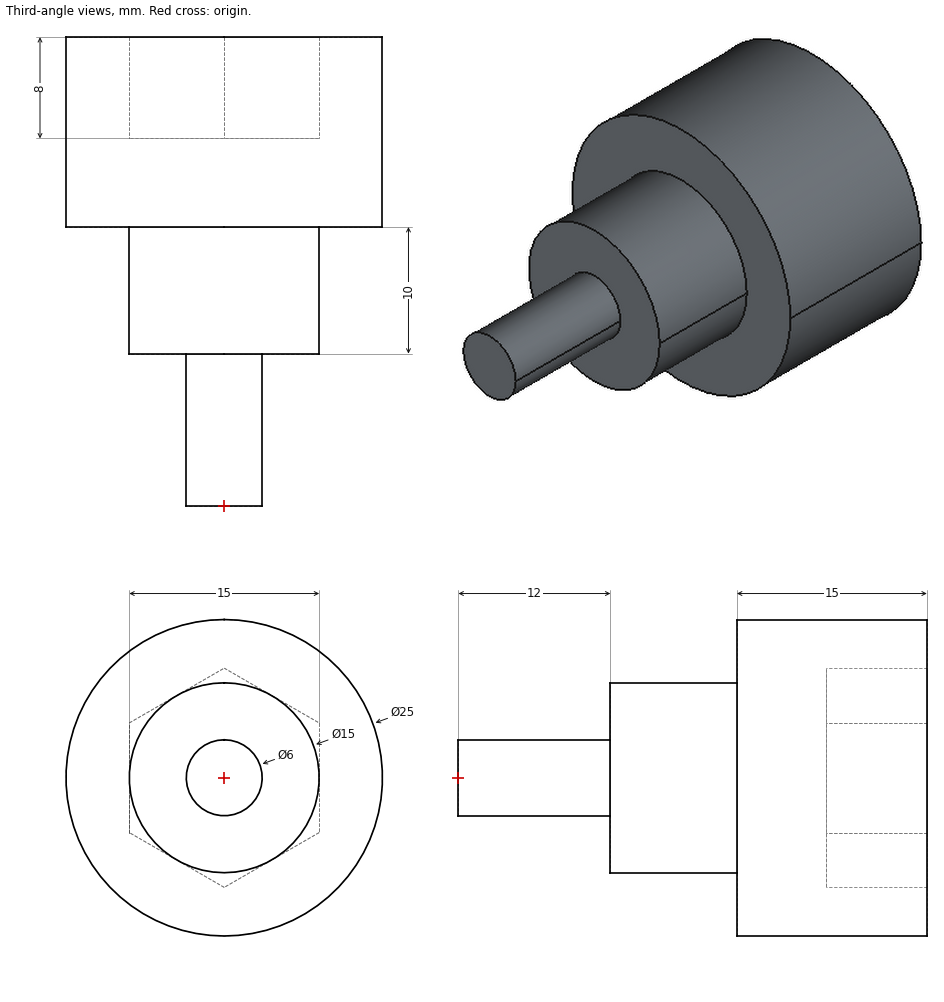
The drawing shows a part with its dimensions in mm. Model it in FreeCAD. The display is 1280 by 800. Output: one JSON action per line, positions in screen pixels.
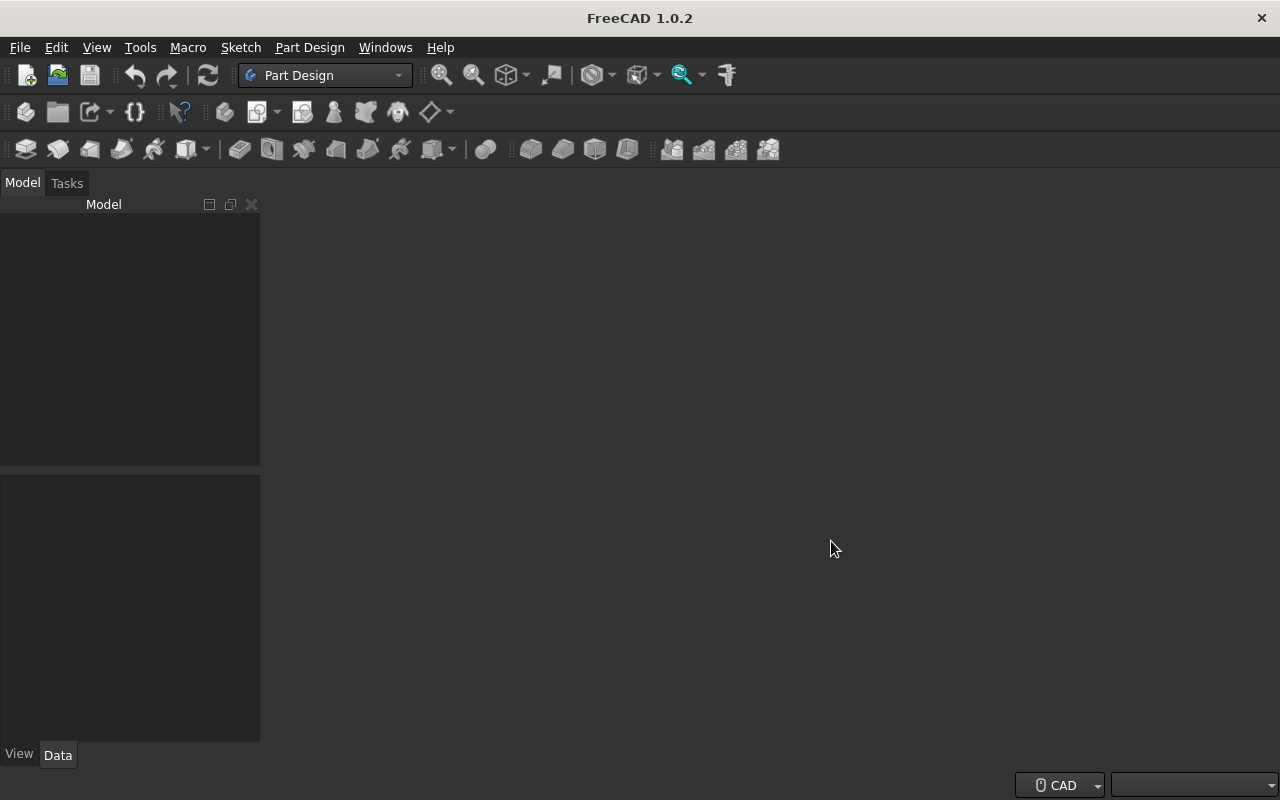
{"action": "key", "text": "ctrl+n"}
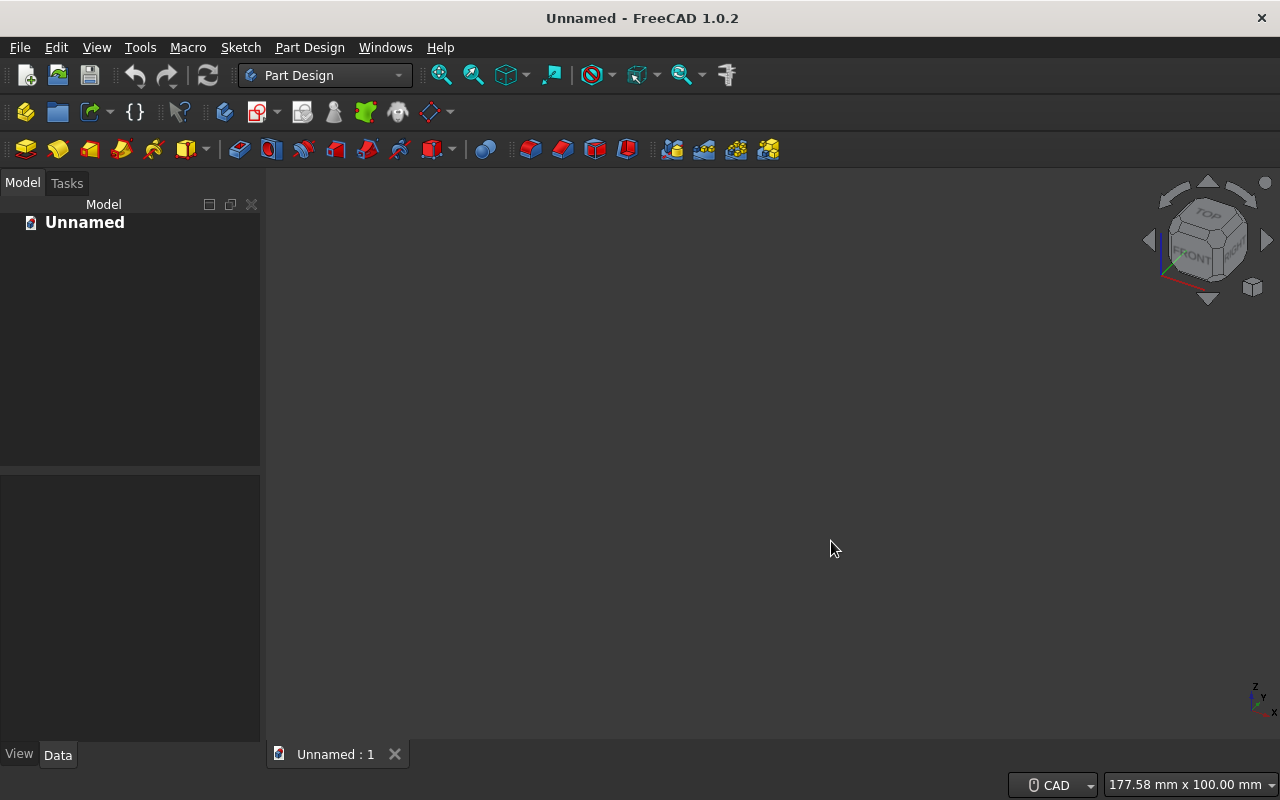
{"action": "left_click", "coordinate": [258, 112]}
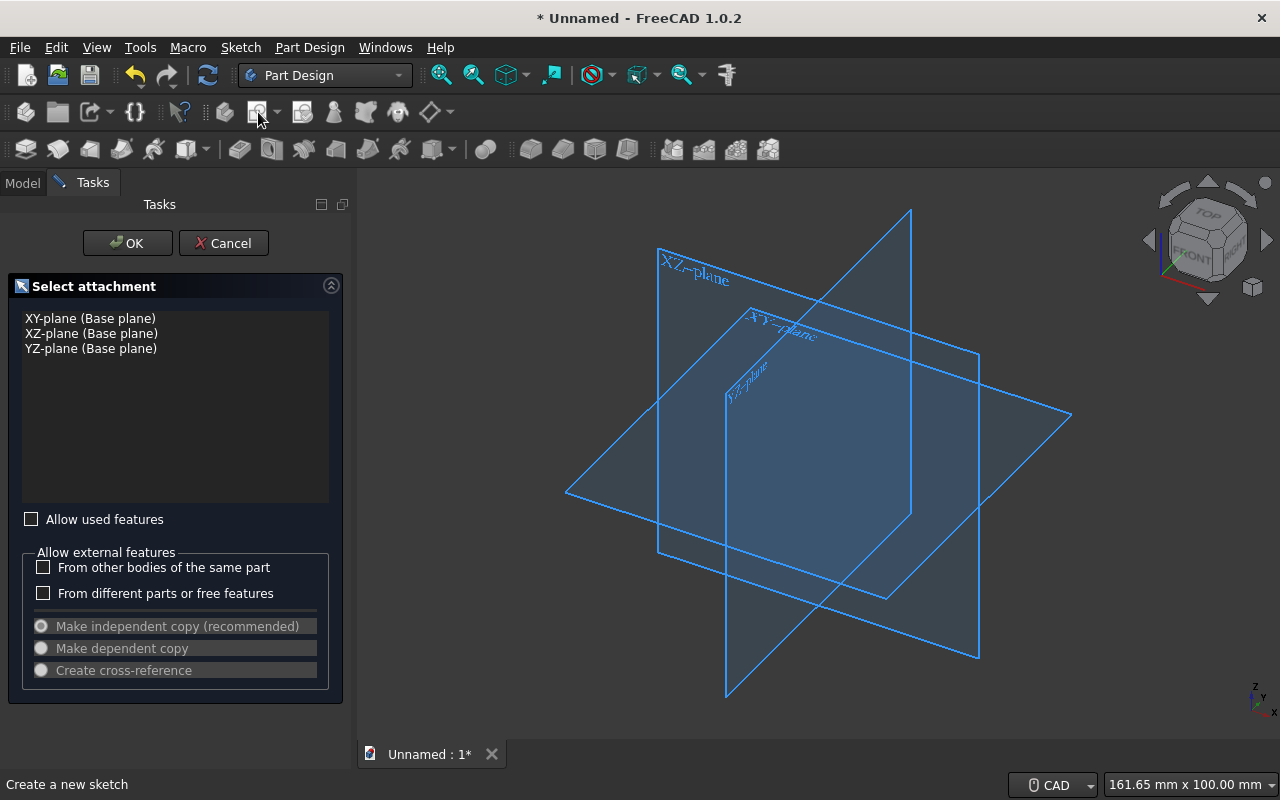
{"action": "left_click", "coordinate": [82, 334]}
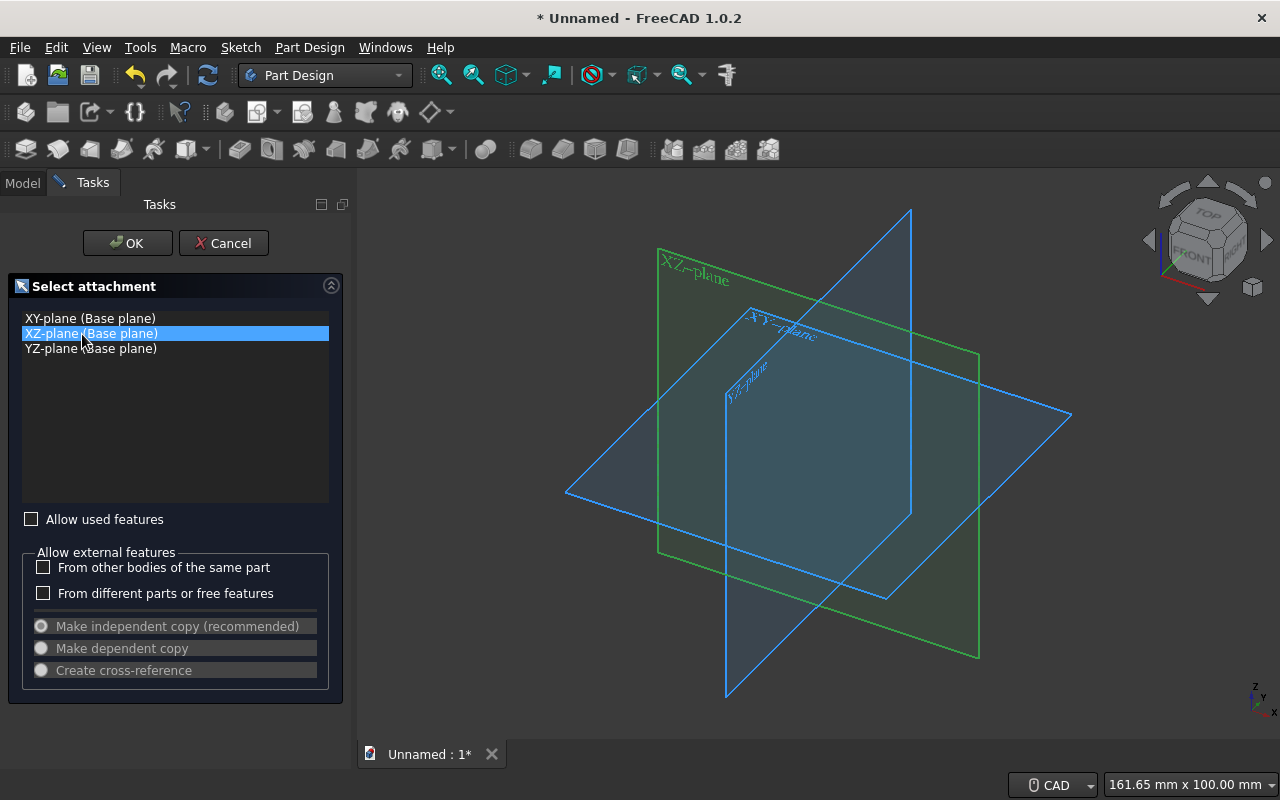
{"action": "left_click", "coordinate": [128, 243]}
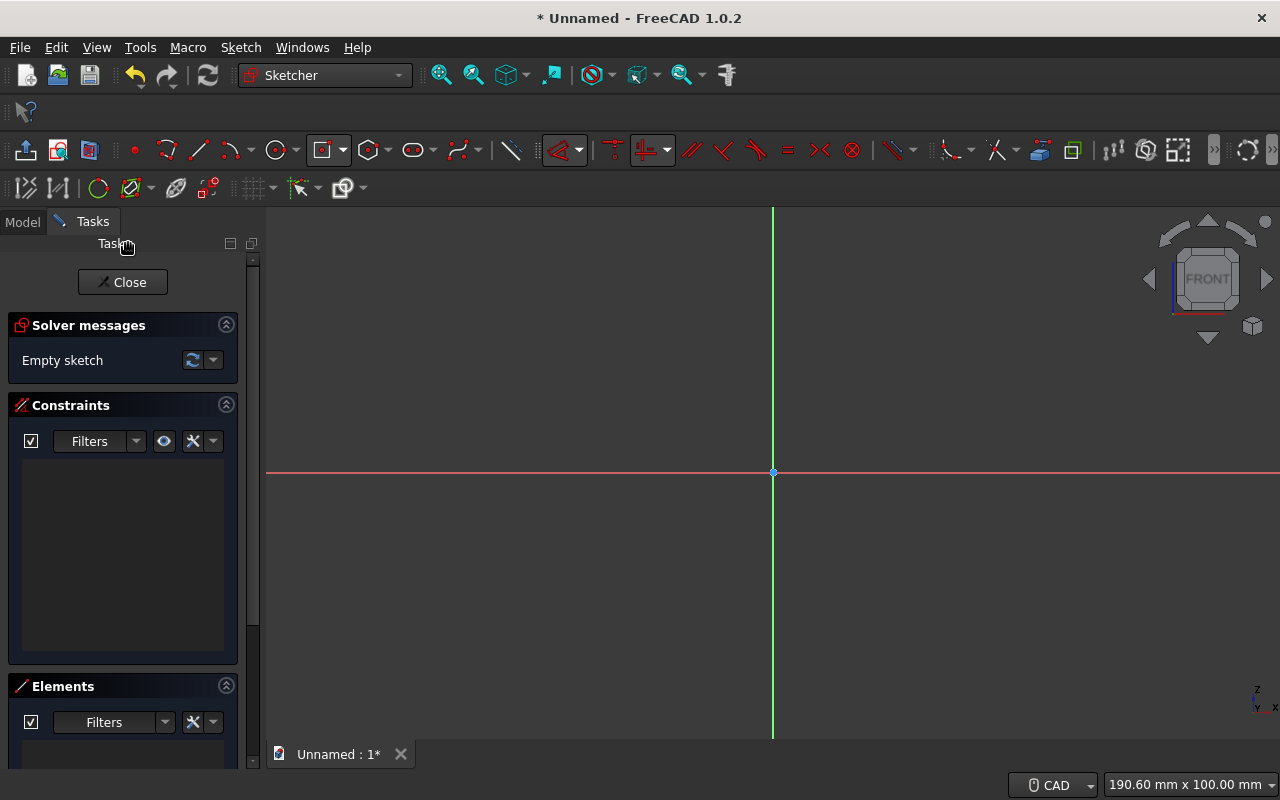
{"action": "scroll", "coordinate": [780, 473], "scroll_direction": "up", "scroll_amount": 12}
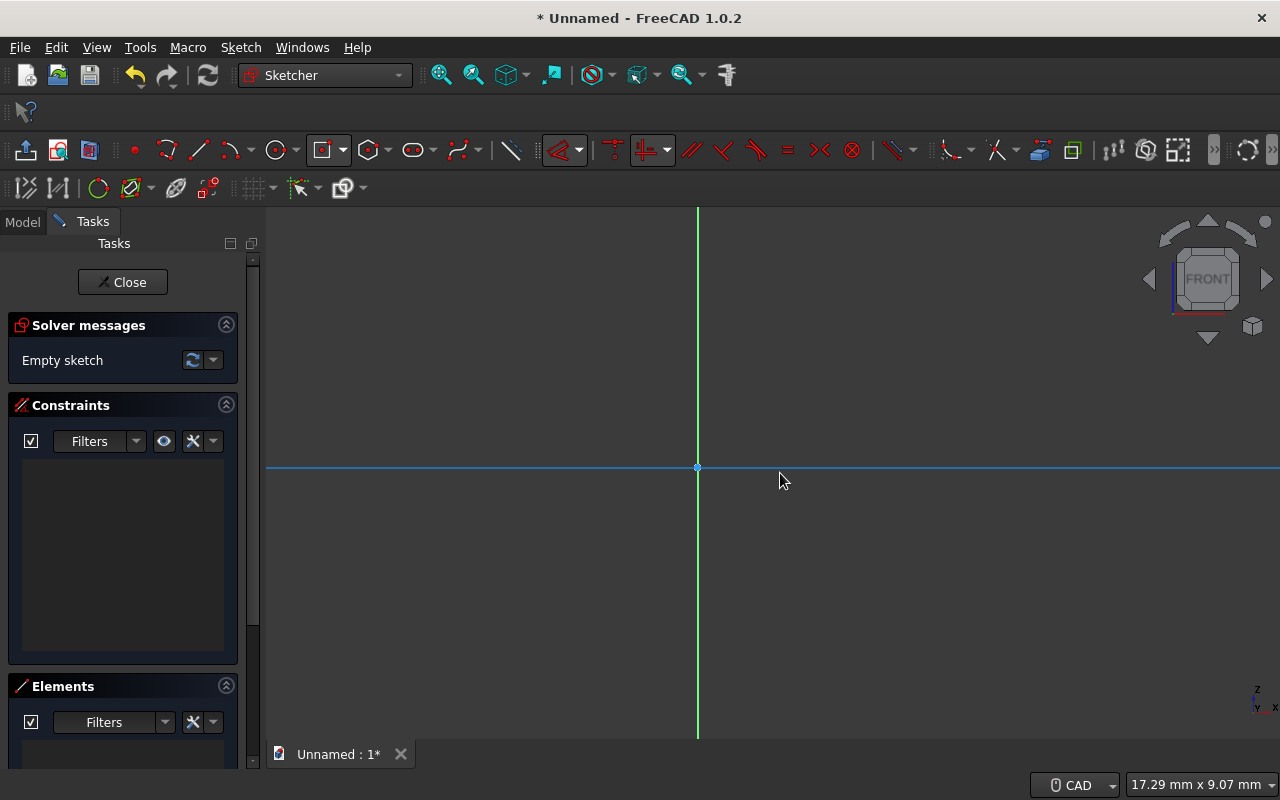
{"action": "key", "text": "g c"}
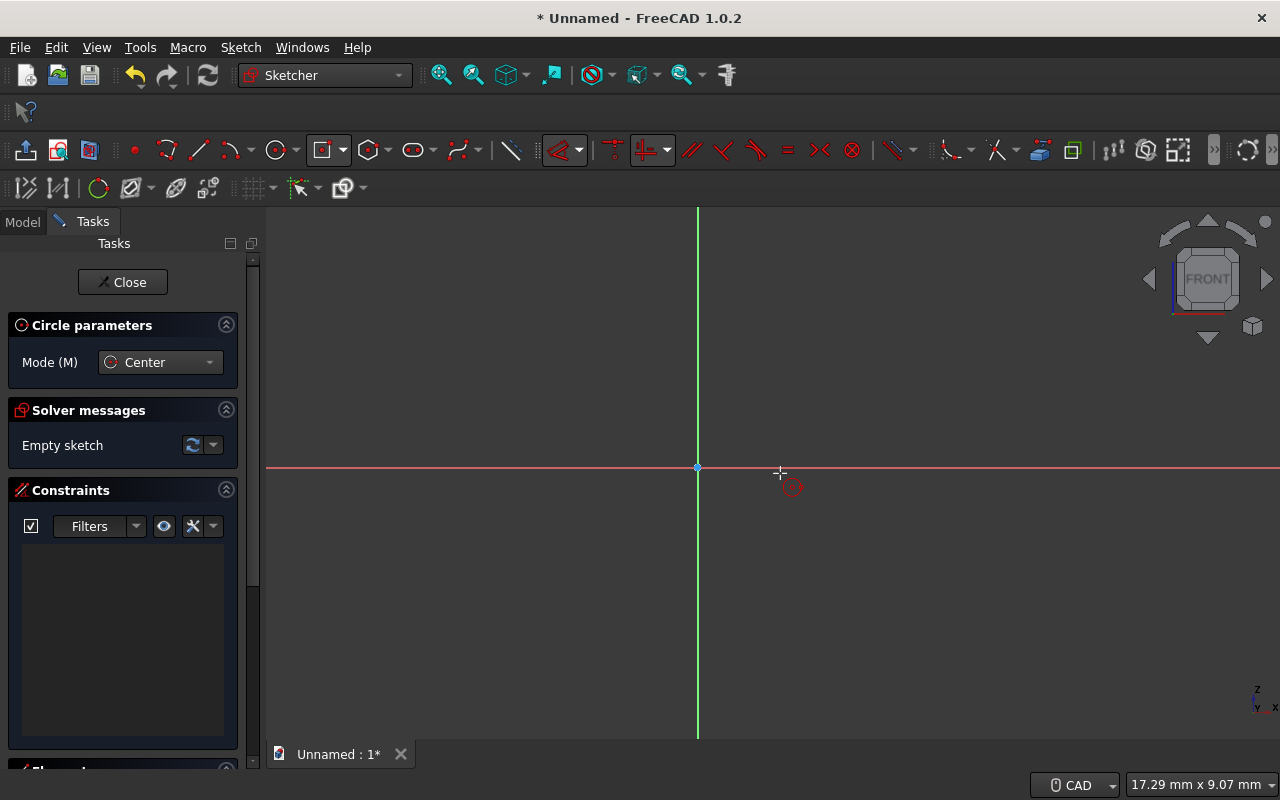
{"action": "left_click", "coordinate": [698, 468]}
{"action": "left_click", "coordinate": [822, 344]}
{"action": "key", "text": "Escape"}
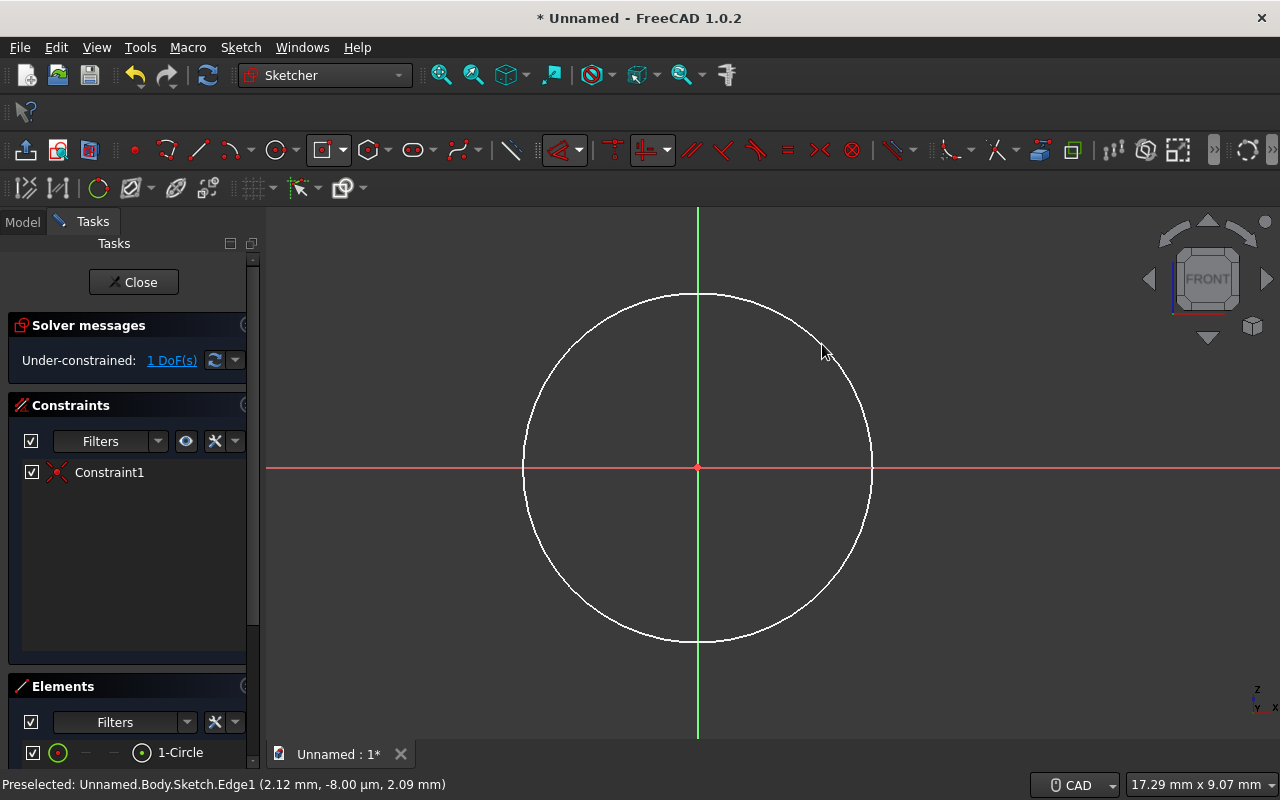
{"action": "left_click", "coordinate": [821, 344]}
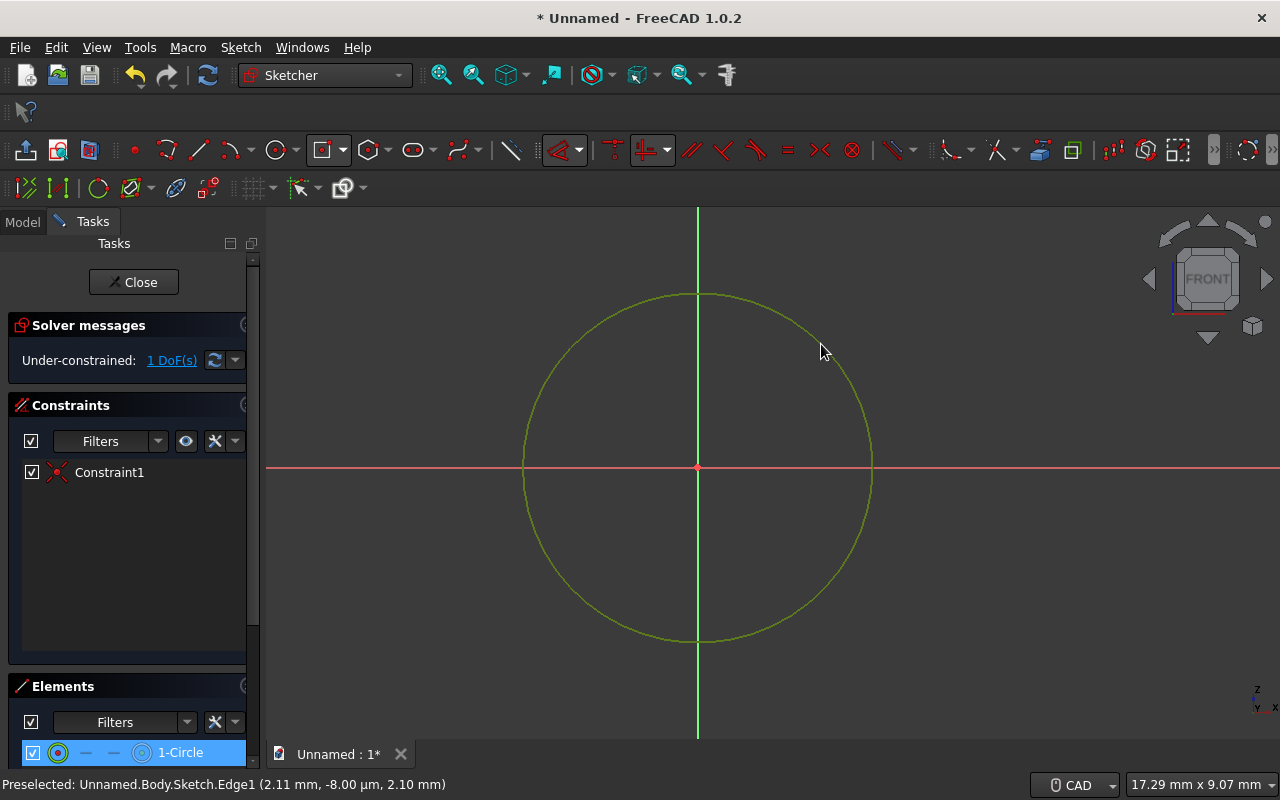
{"action": "key", "text": "k o"}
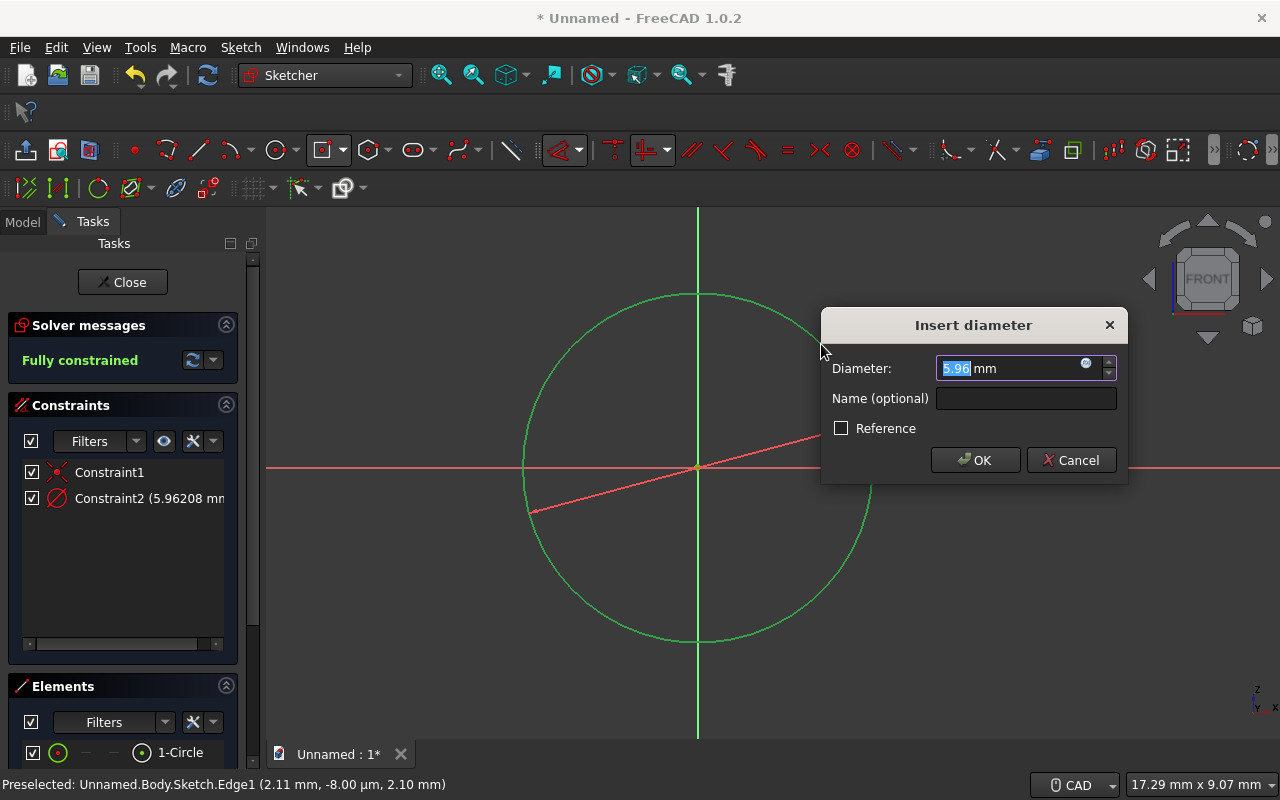
{"action": "type", "text": "6"}
{"action": "key", "text": "Return"}